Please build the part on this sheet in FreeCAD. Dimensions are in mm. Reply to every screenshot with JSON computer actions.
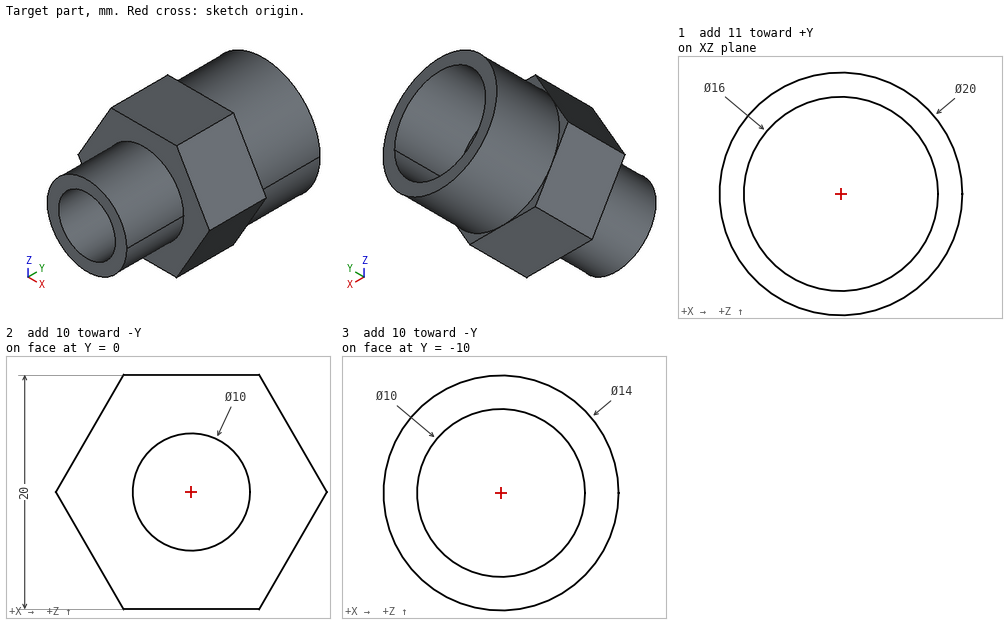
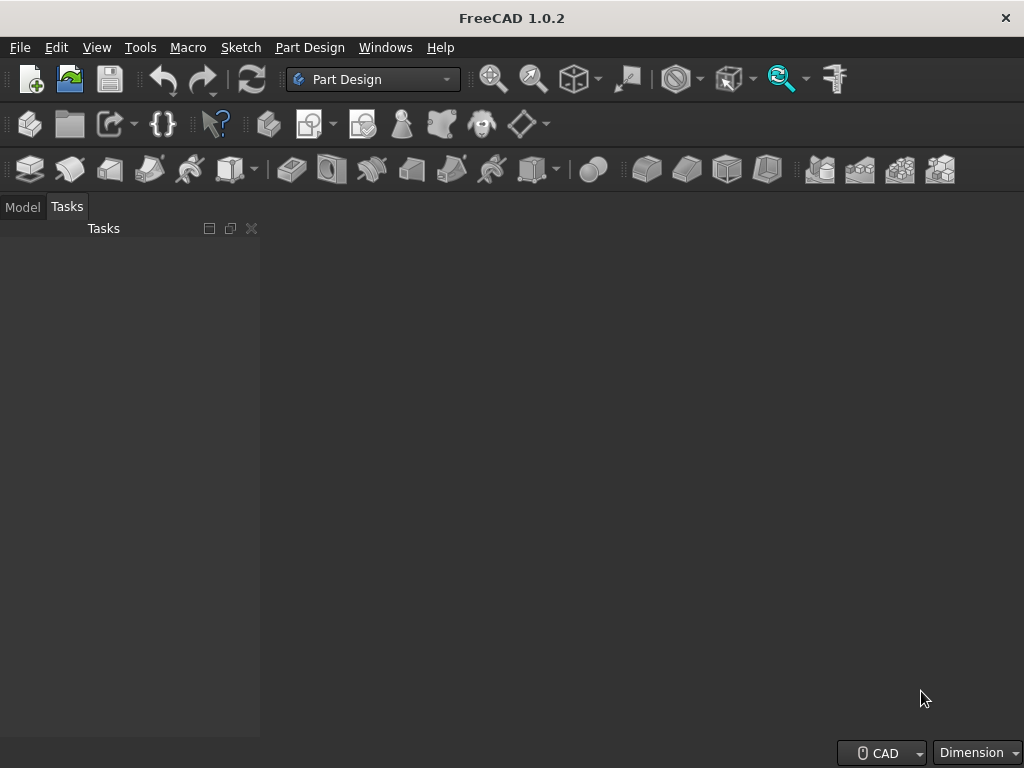
{"action": "left_click", "coordinate": [30, 80]}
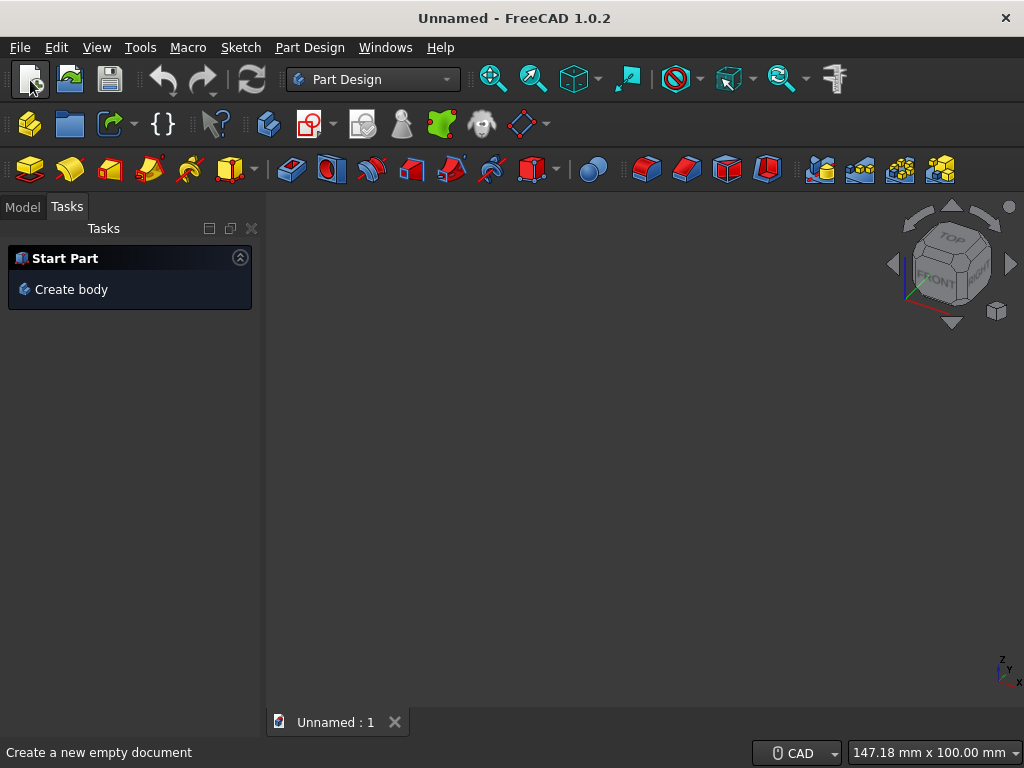
{"action": "left_click", "coordinate": [310, 124]}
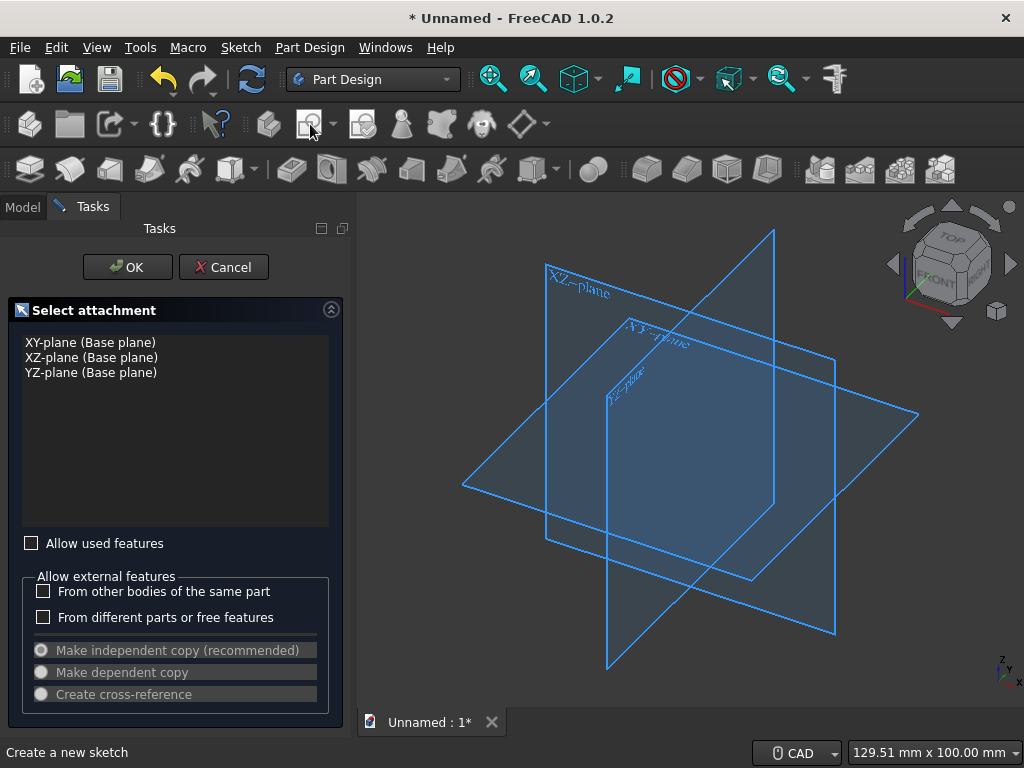
{"action": "left_click", "coordinate": [82, 358]}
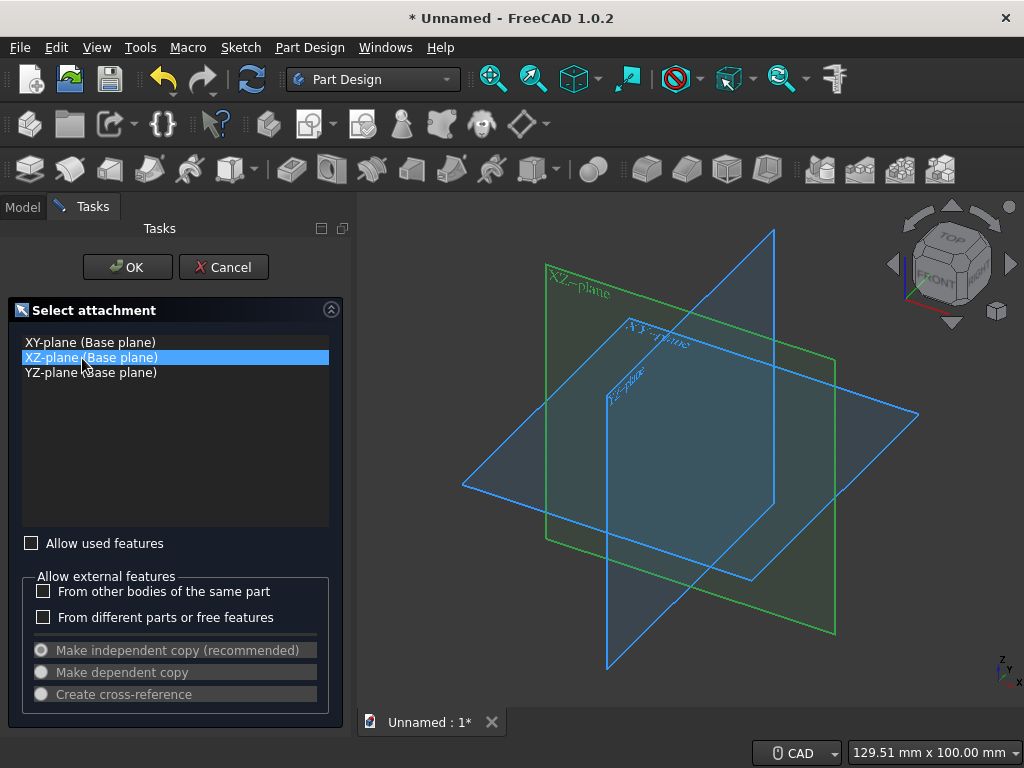
{"action": "left_click", "coordinate": [128, 267]}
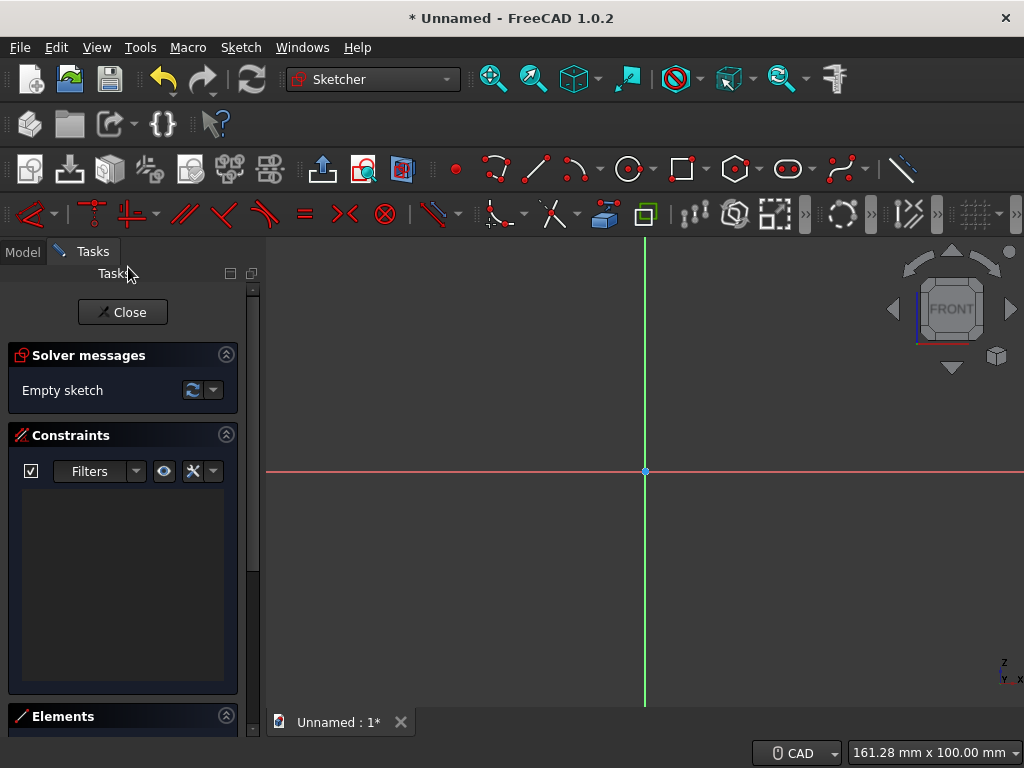
{"action": "scroll", "coordinate": [675, 472], "scroll_direction": "up", "scroll_amount": 6}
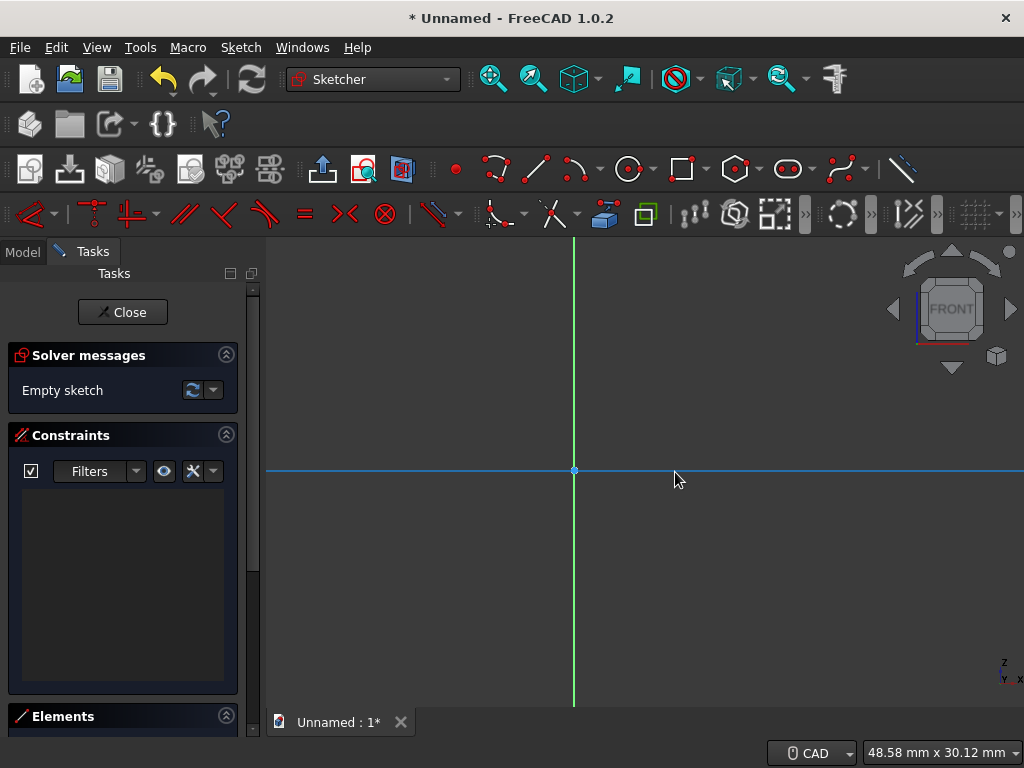
{"action": "left_click", "coordinate": [630, 170]}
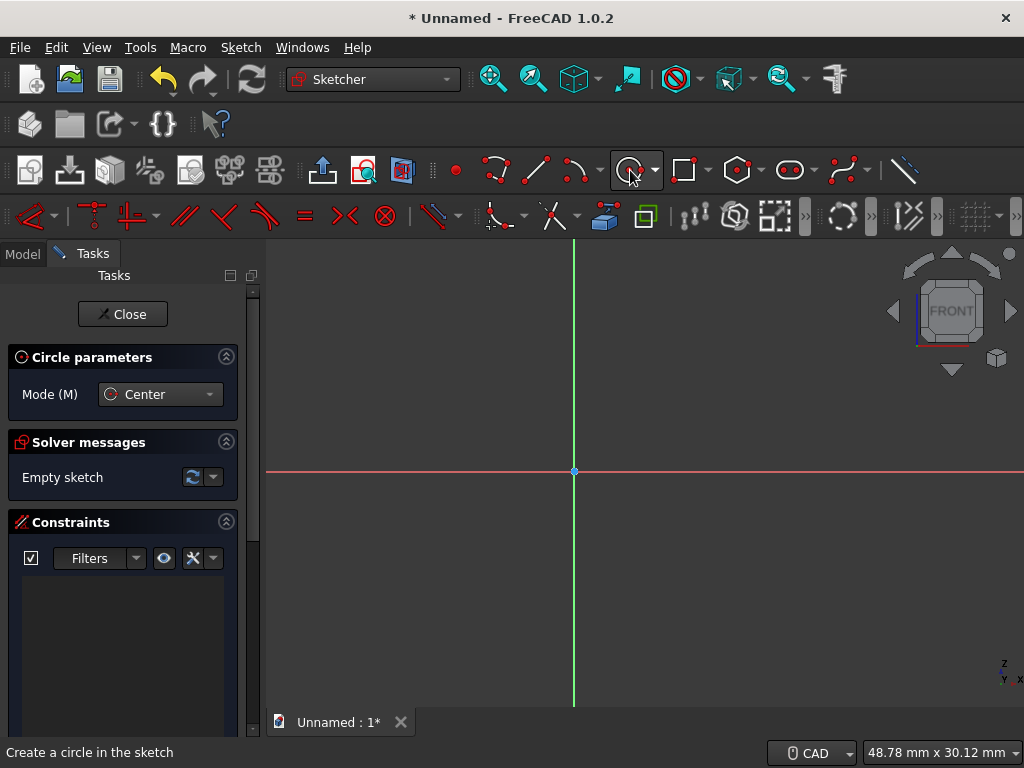
{"action": "left_click", "coordinate": [574, 472]}
{"action": "left_click", "coordinate": [684, 362]}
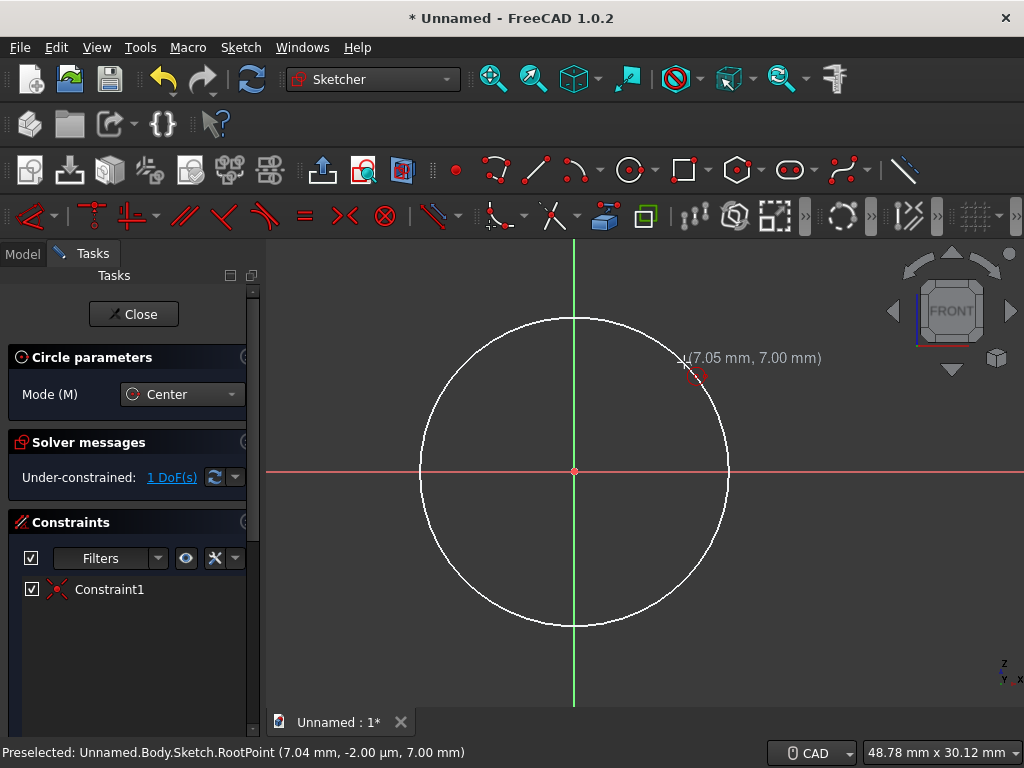
{"action": "left_click", "coordinate": [574, 472]}
{"action": "left_click", "coordinate": [662, 384]}
{"action": "key", "text": "Escape"}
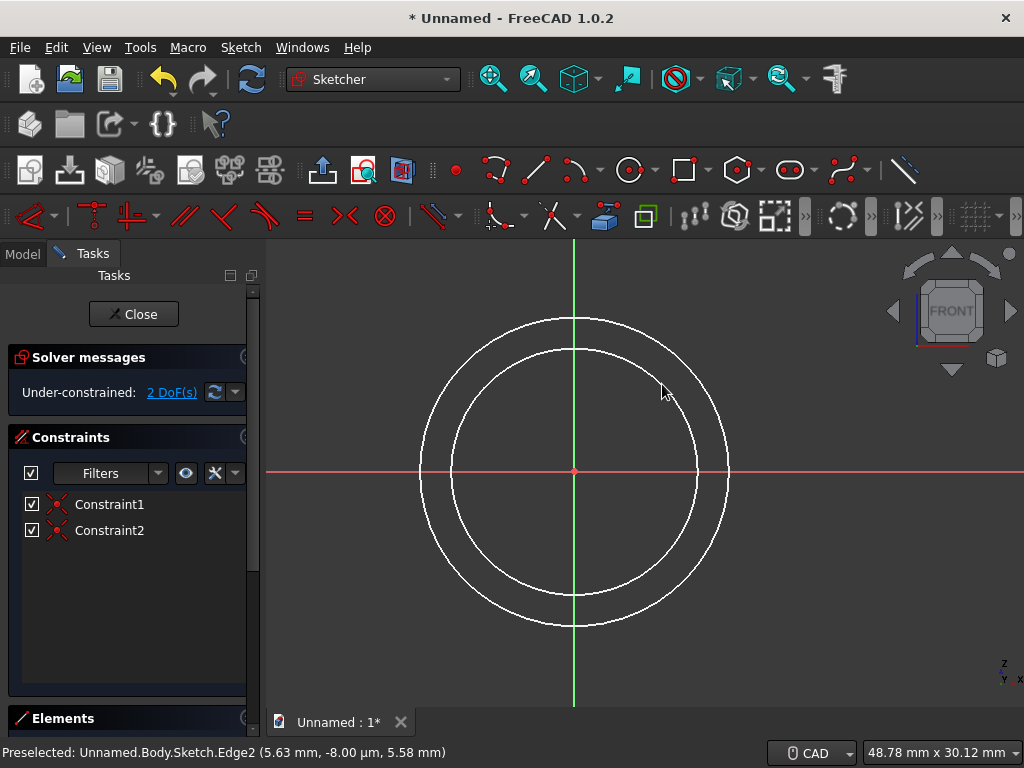
{"action": "left_click", "coordinate": [30, 216]}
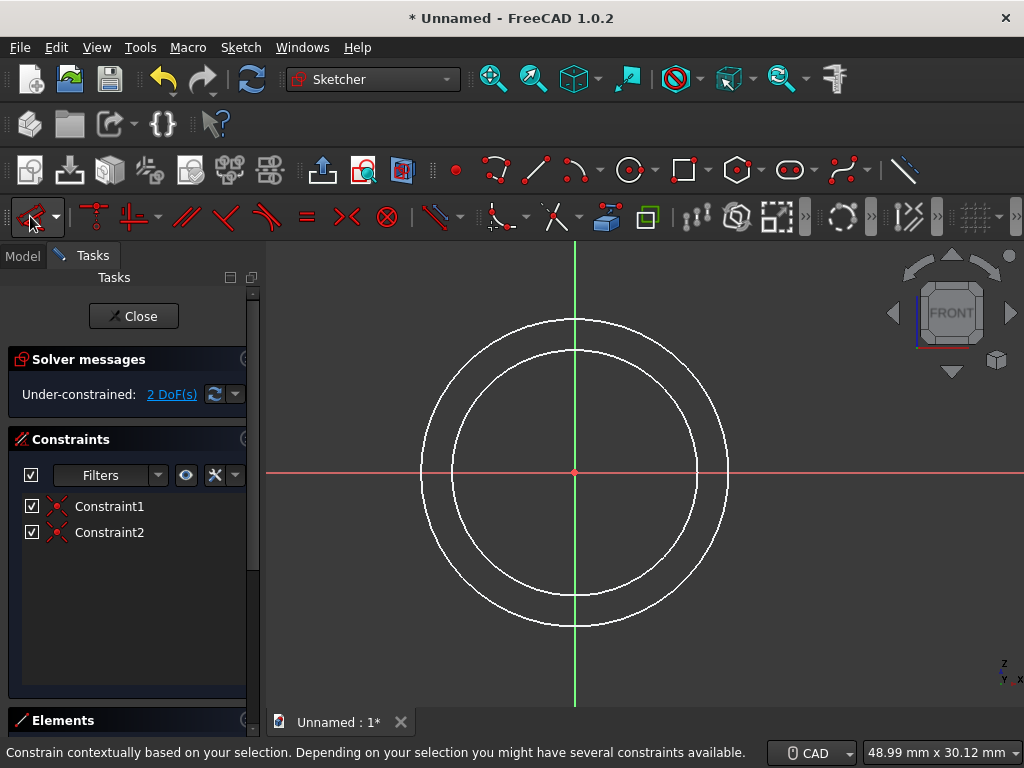
{"action": "left_click", "coordinate": [683, 364]}
{"action": "left_click", "coordinate": [706, 341]}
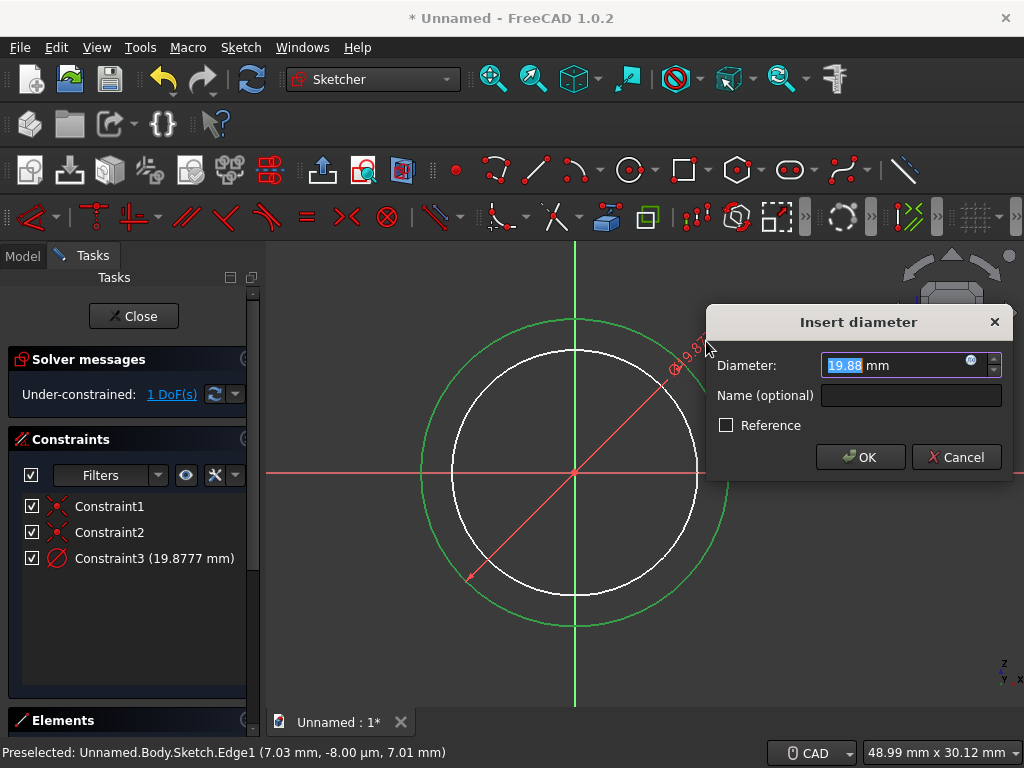
{"action": "type", "text": "20"}
{"action": "key", "text": "Return"}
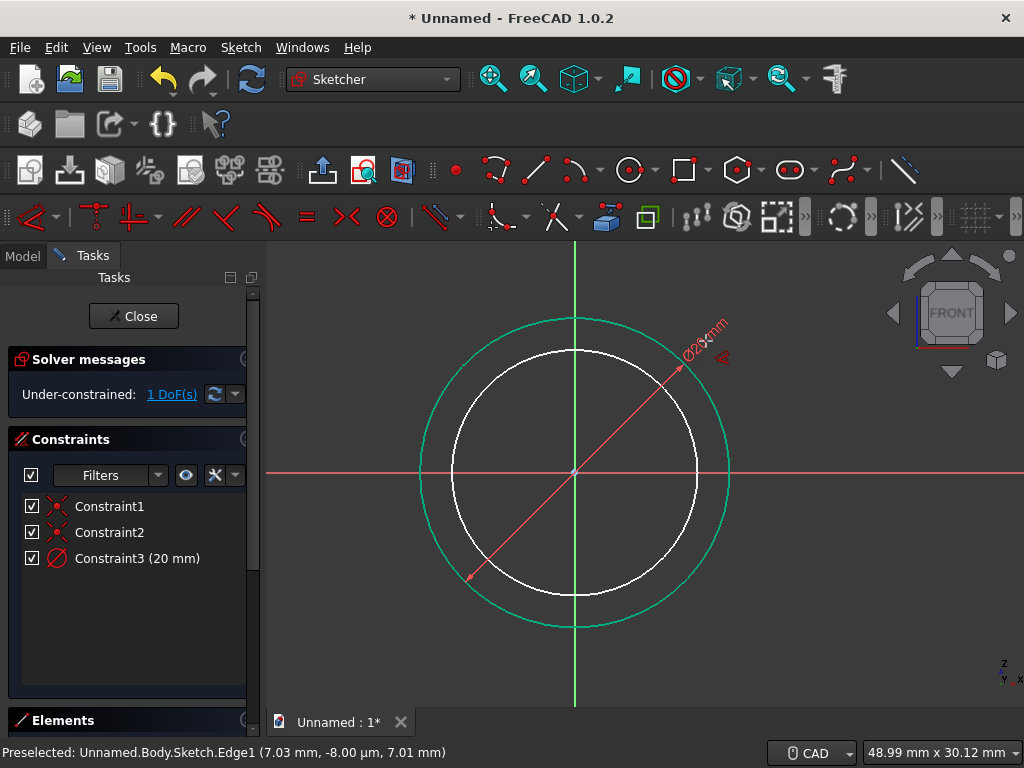
{"action": "left_click", "coordinate": [661, 386]}
{"action": "left_click", "coordinate": [745, 422]}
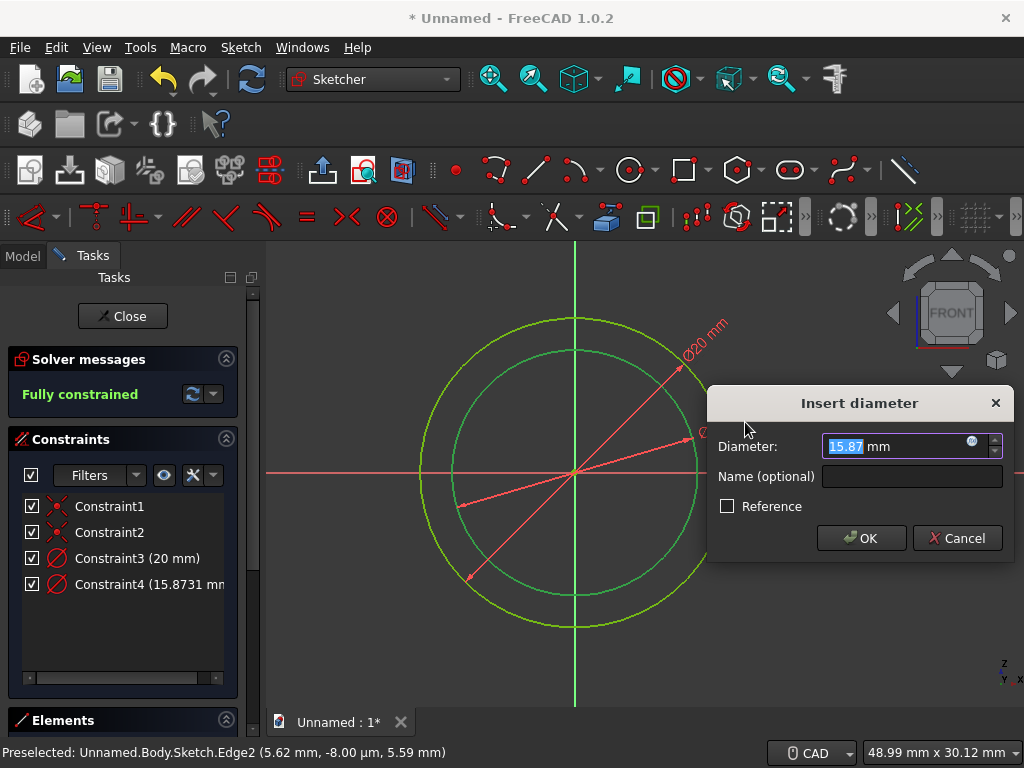
{"action": "type", "text": "16"}
{"action": "key", "text": "Return"}
{"action": "key", "text": "Escape"}